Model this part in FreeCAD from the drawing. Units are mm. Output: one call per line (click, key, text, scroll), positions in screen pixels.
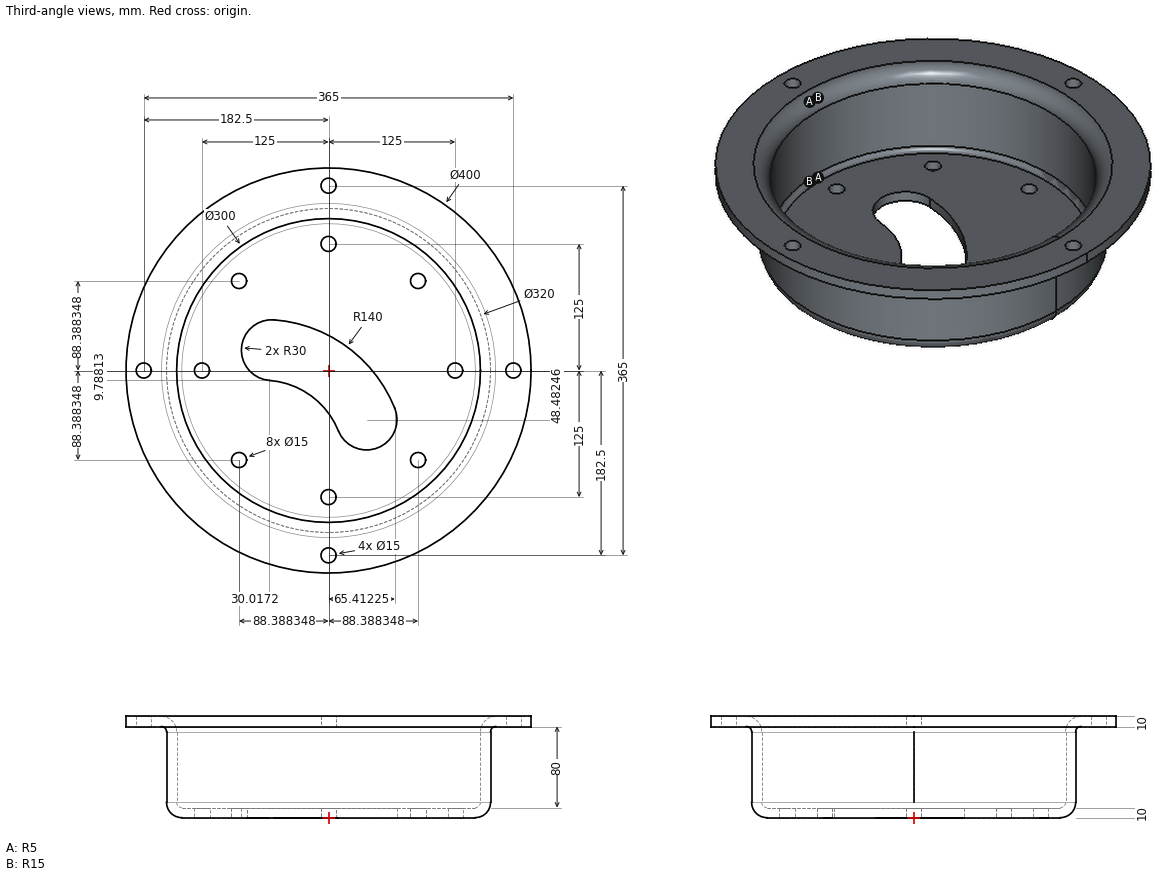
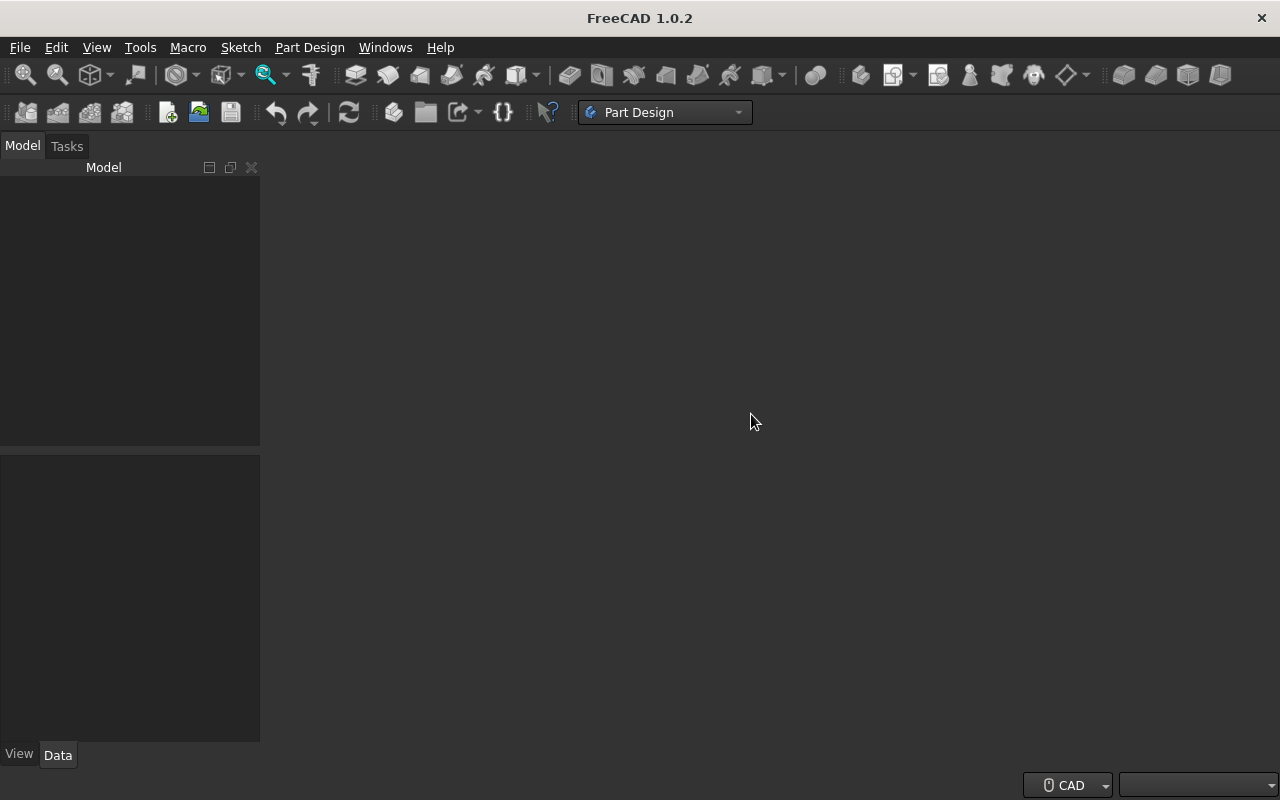
click(168, 112)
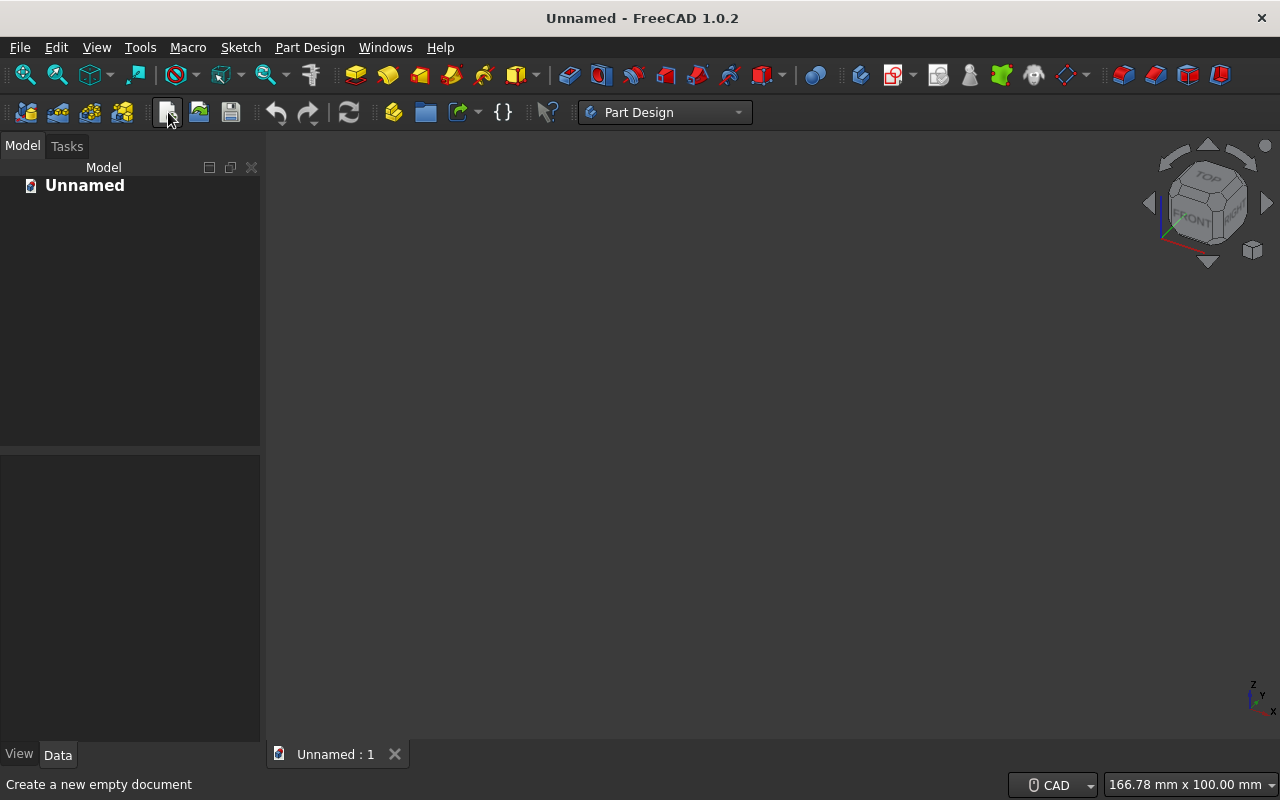
click(894, 76)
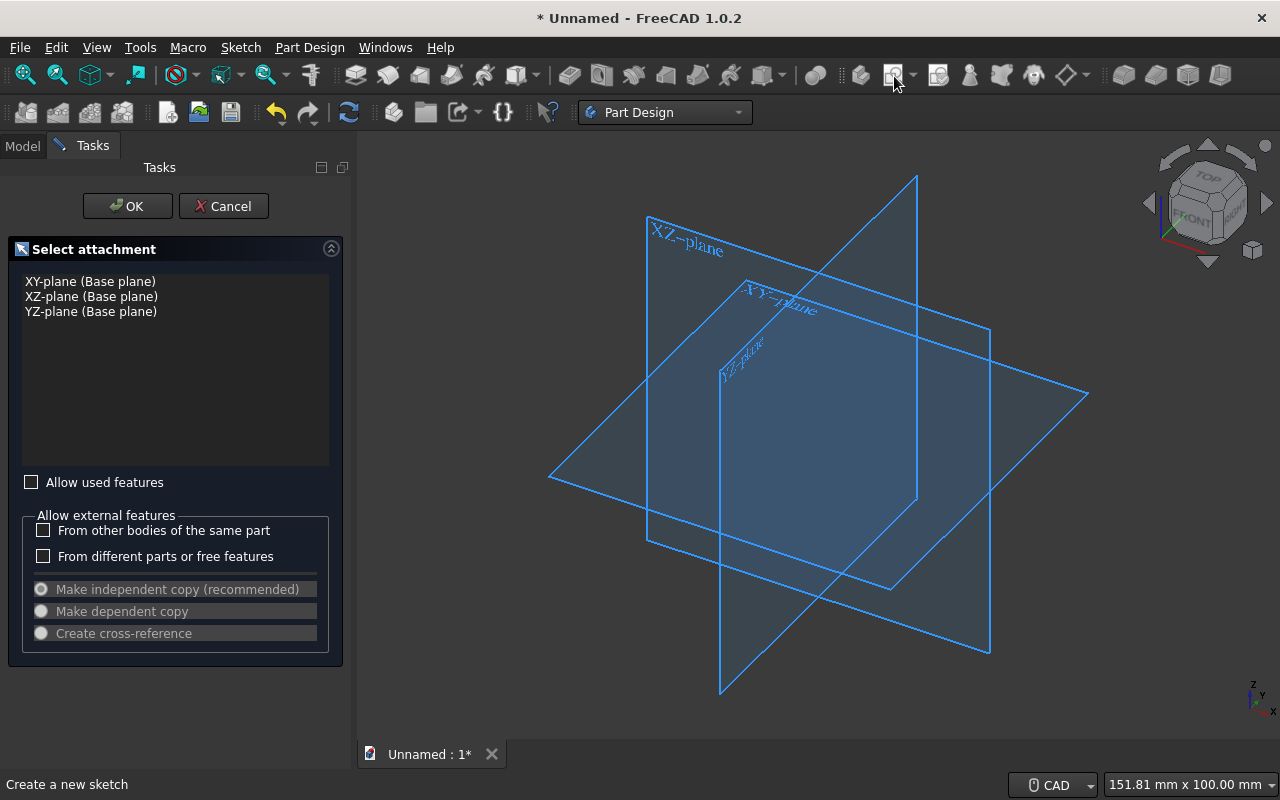
click(82, 282)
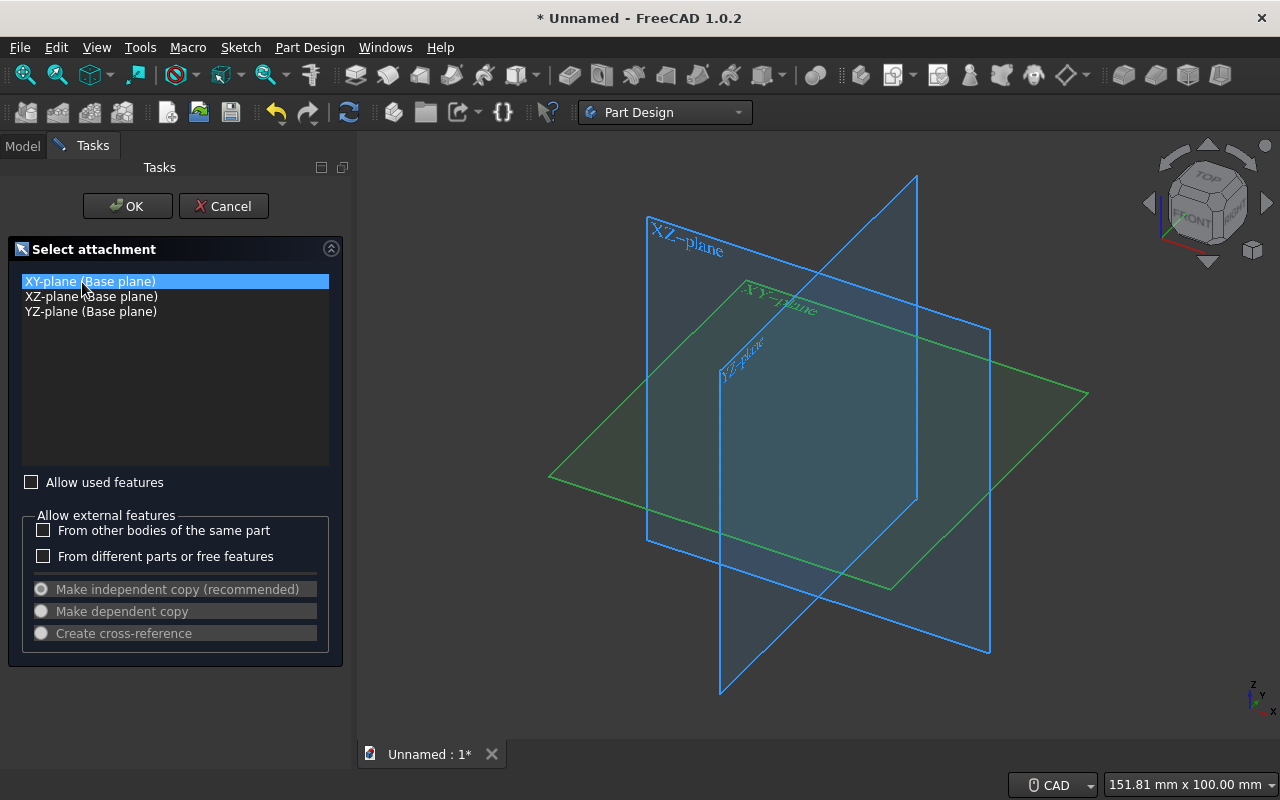
click(128, 206)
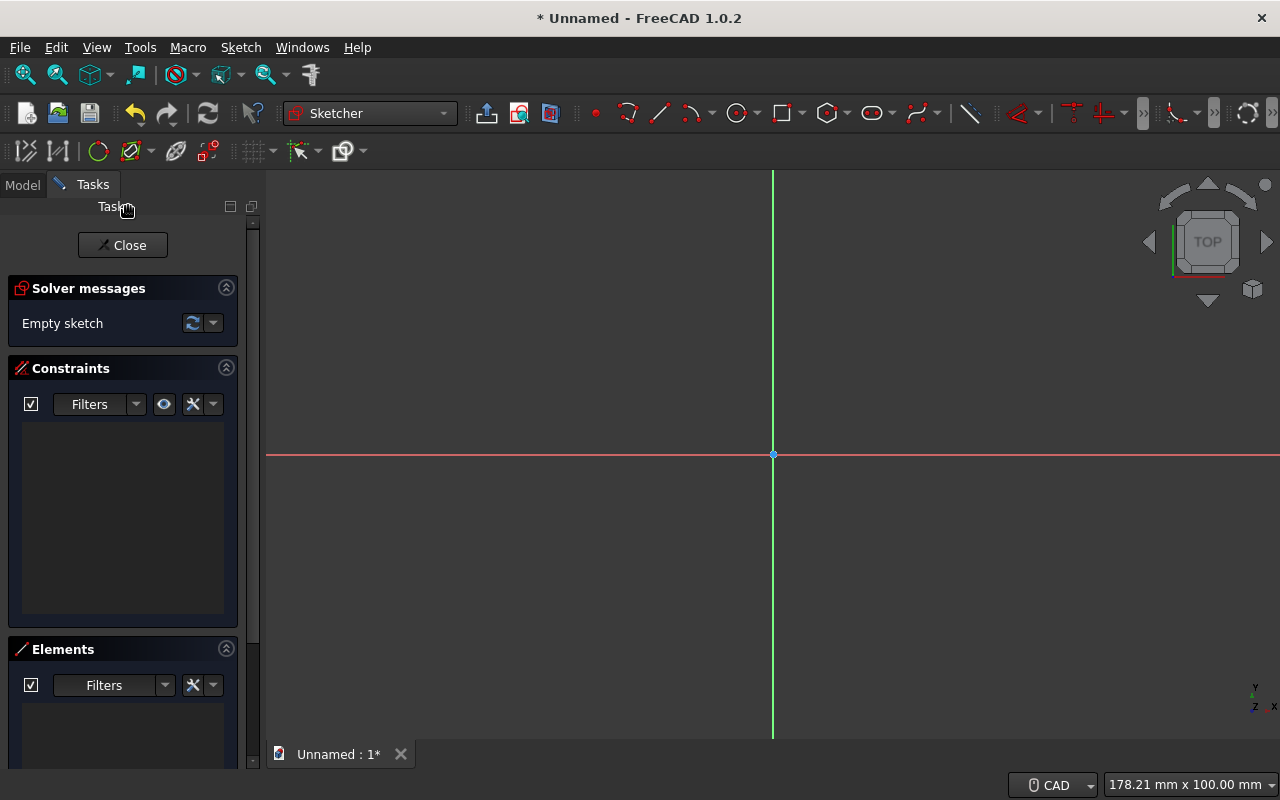
scroll(687, 454, down, 8)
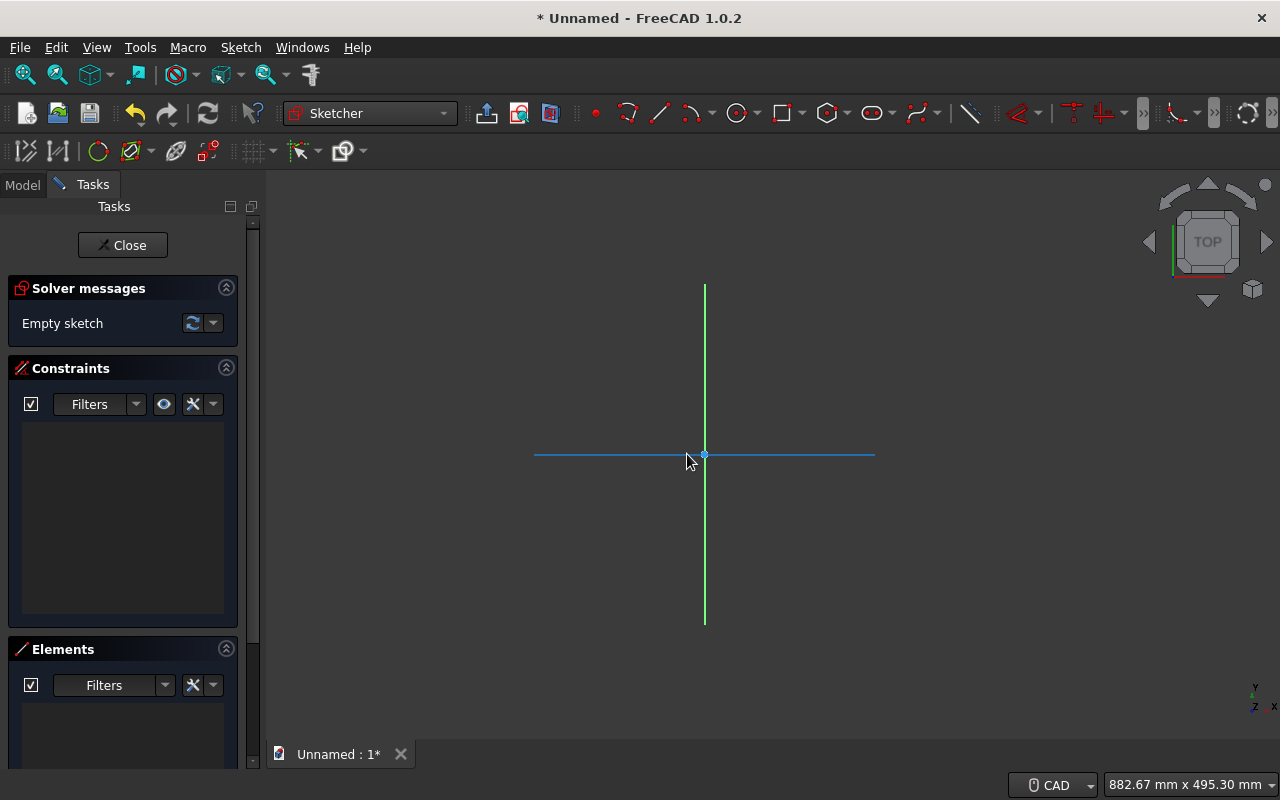
click(714, 114)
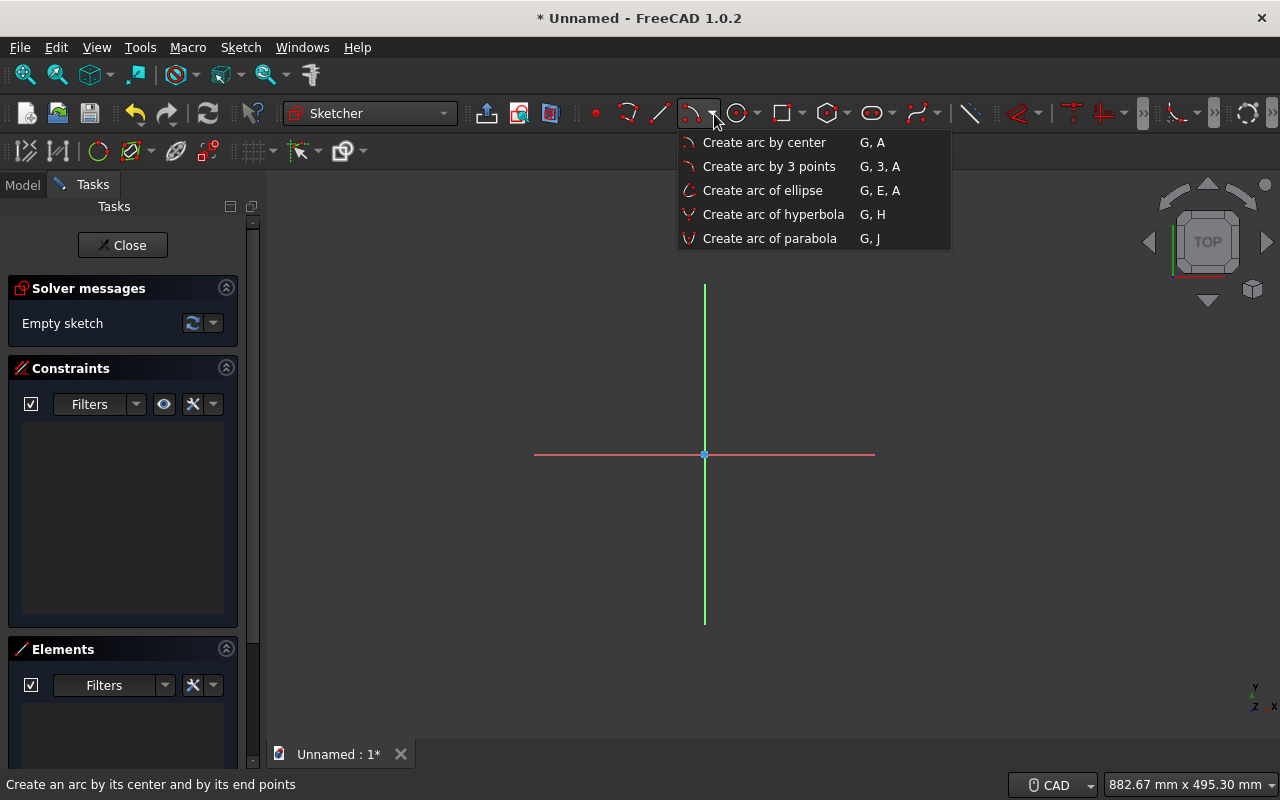
click(814, 166)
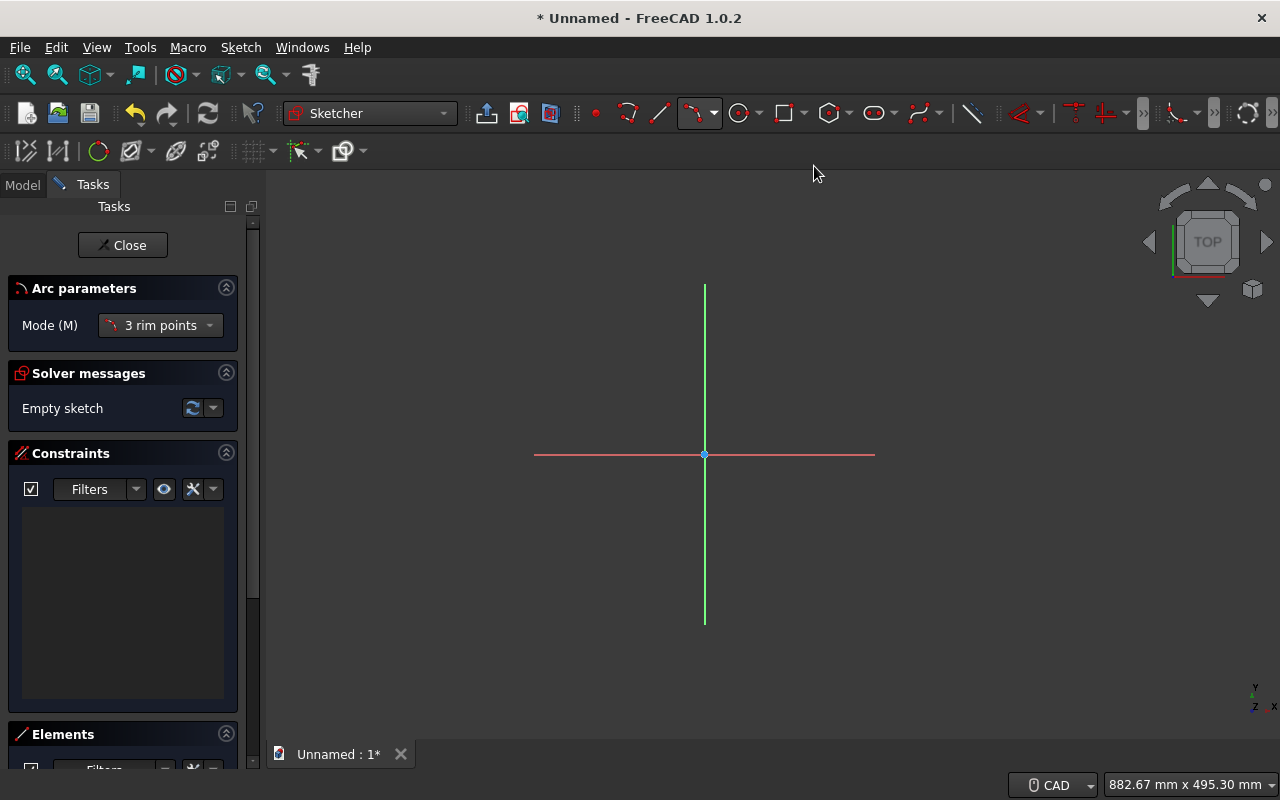
scroll(638, 466, up, 2)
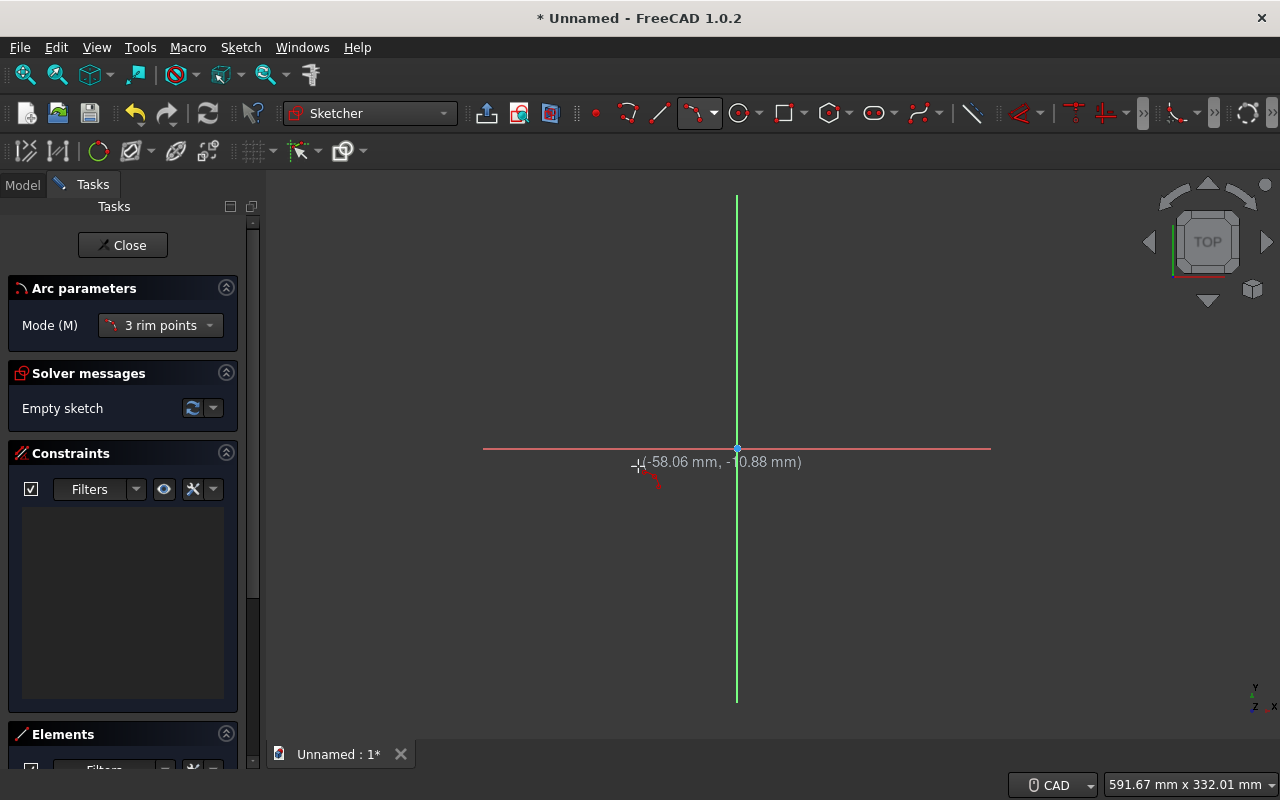
click(637, 465)
click(645, 363)
click(590, 410)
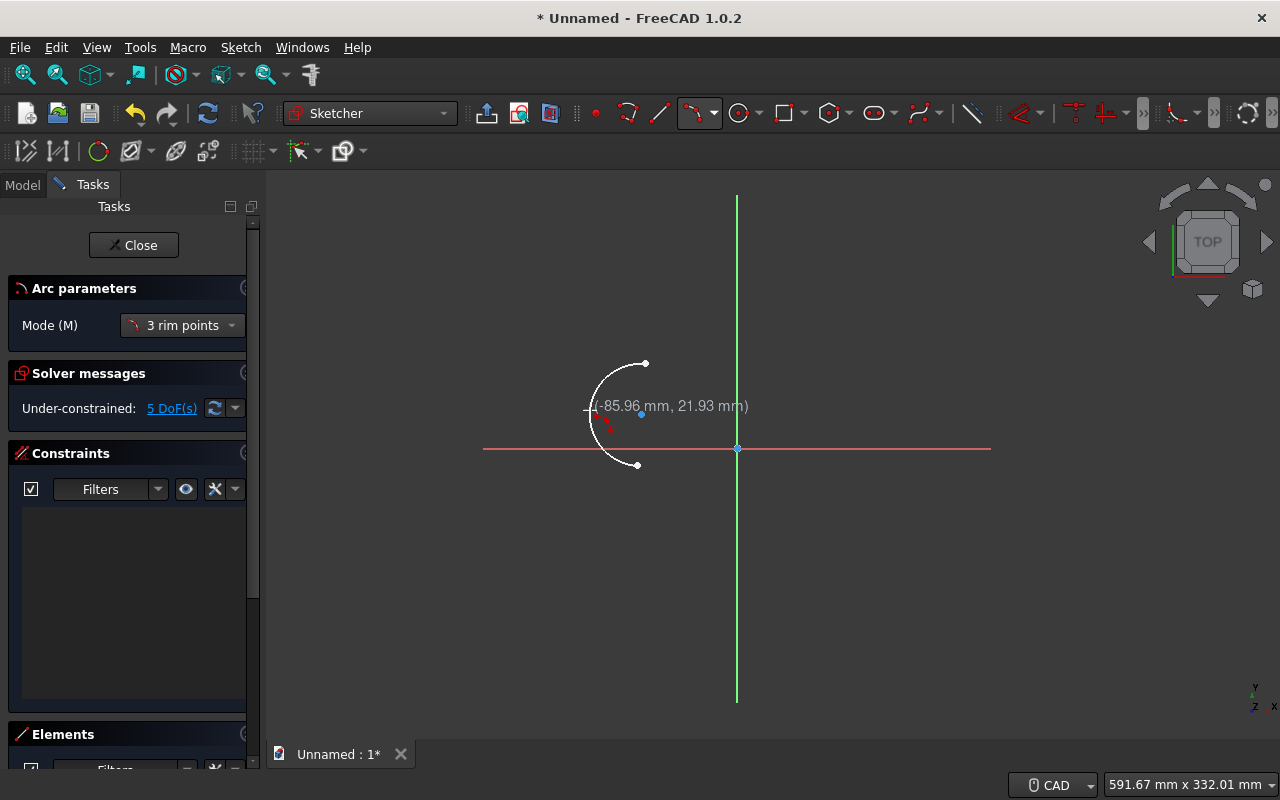
click(645, 364)
click(849, 512)
click(769, 409)